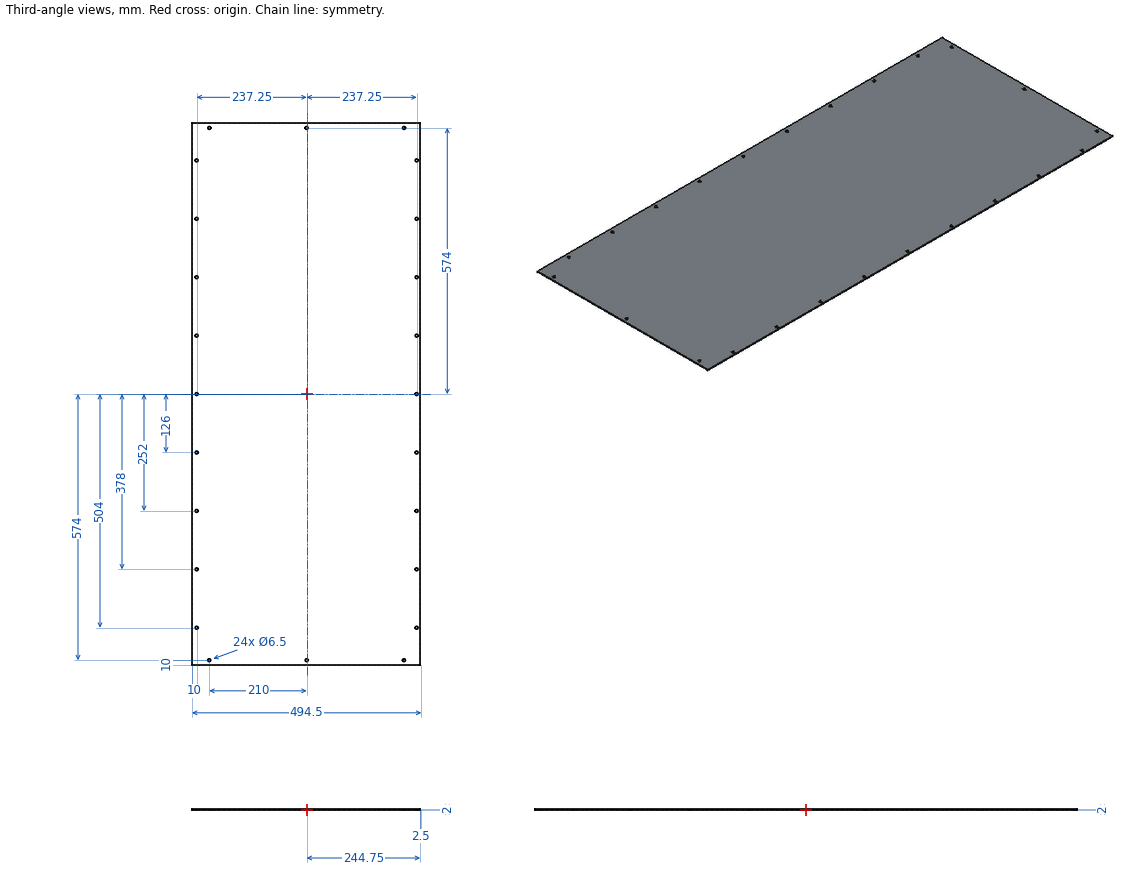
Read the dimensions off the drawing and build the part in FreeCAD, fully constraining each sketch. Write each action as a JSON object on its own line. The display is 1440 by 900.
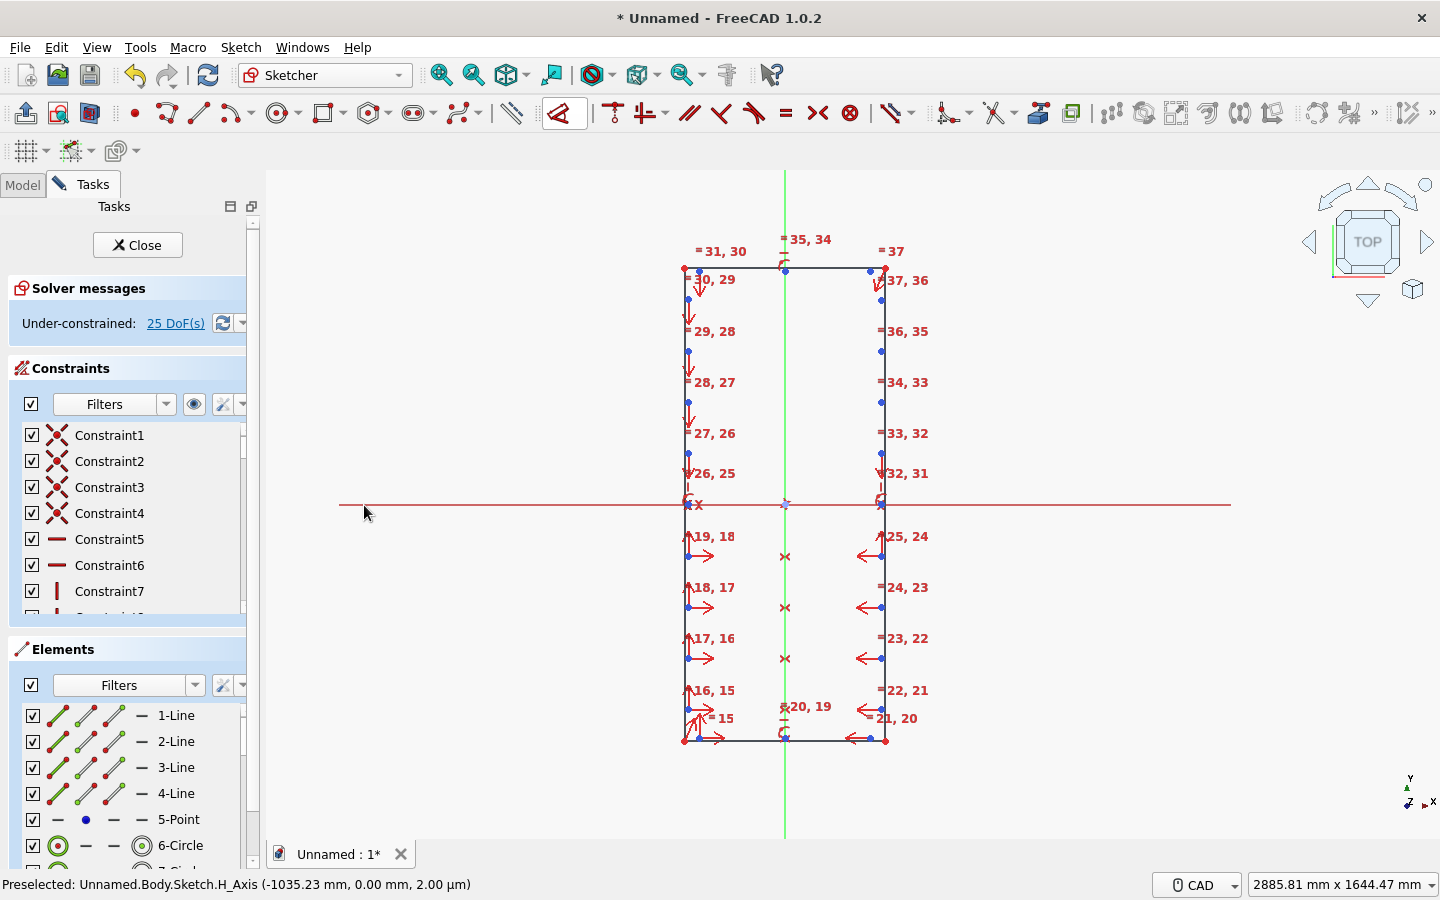
{"action": "left_click", "coordinate": [882, 608]}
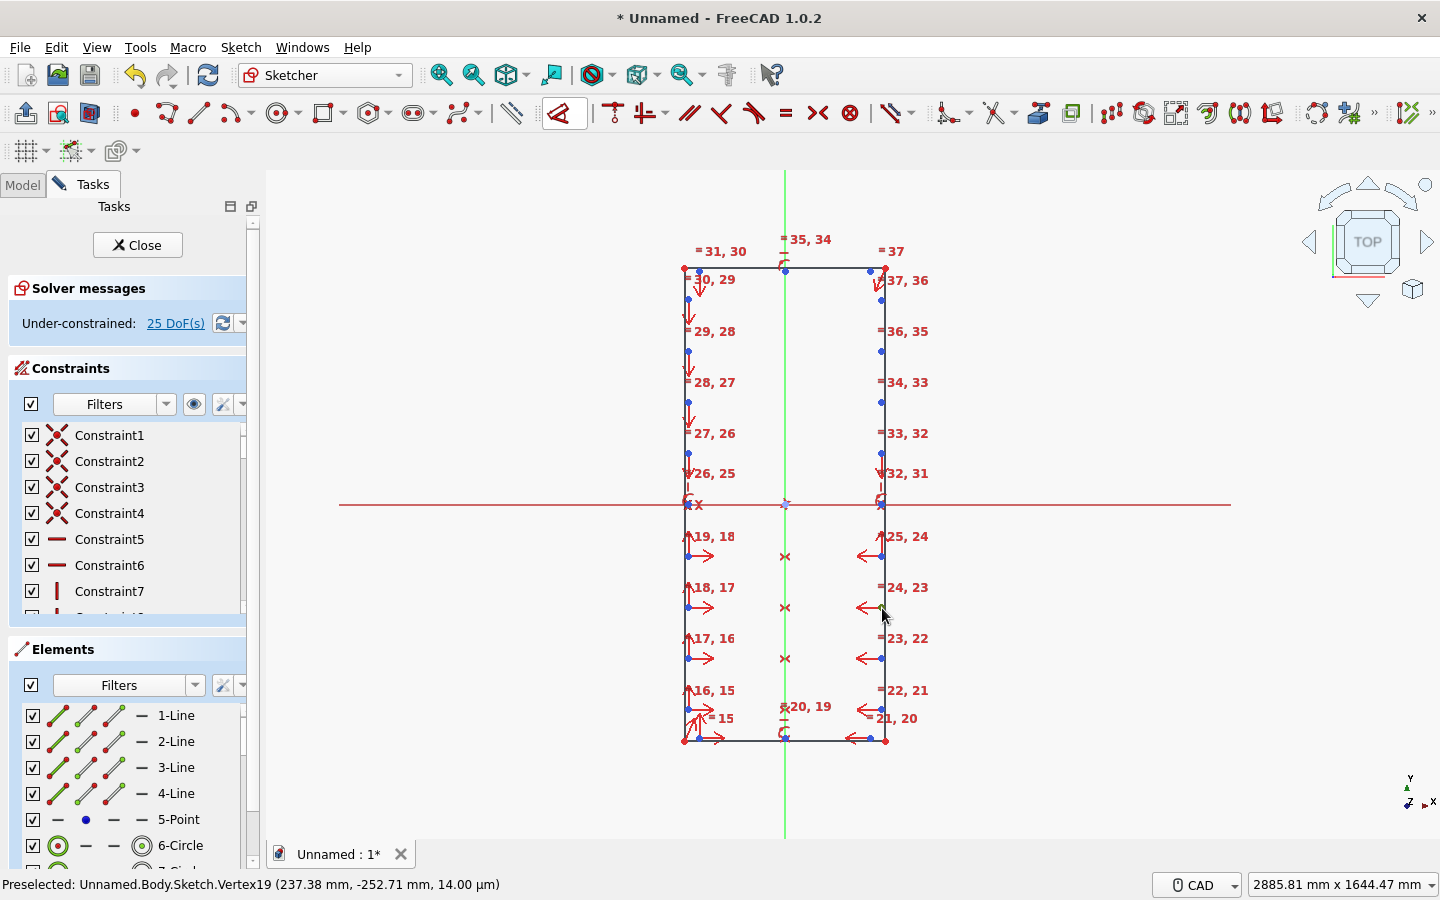
{"action": "left_click", "coordinate": [882, 403]}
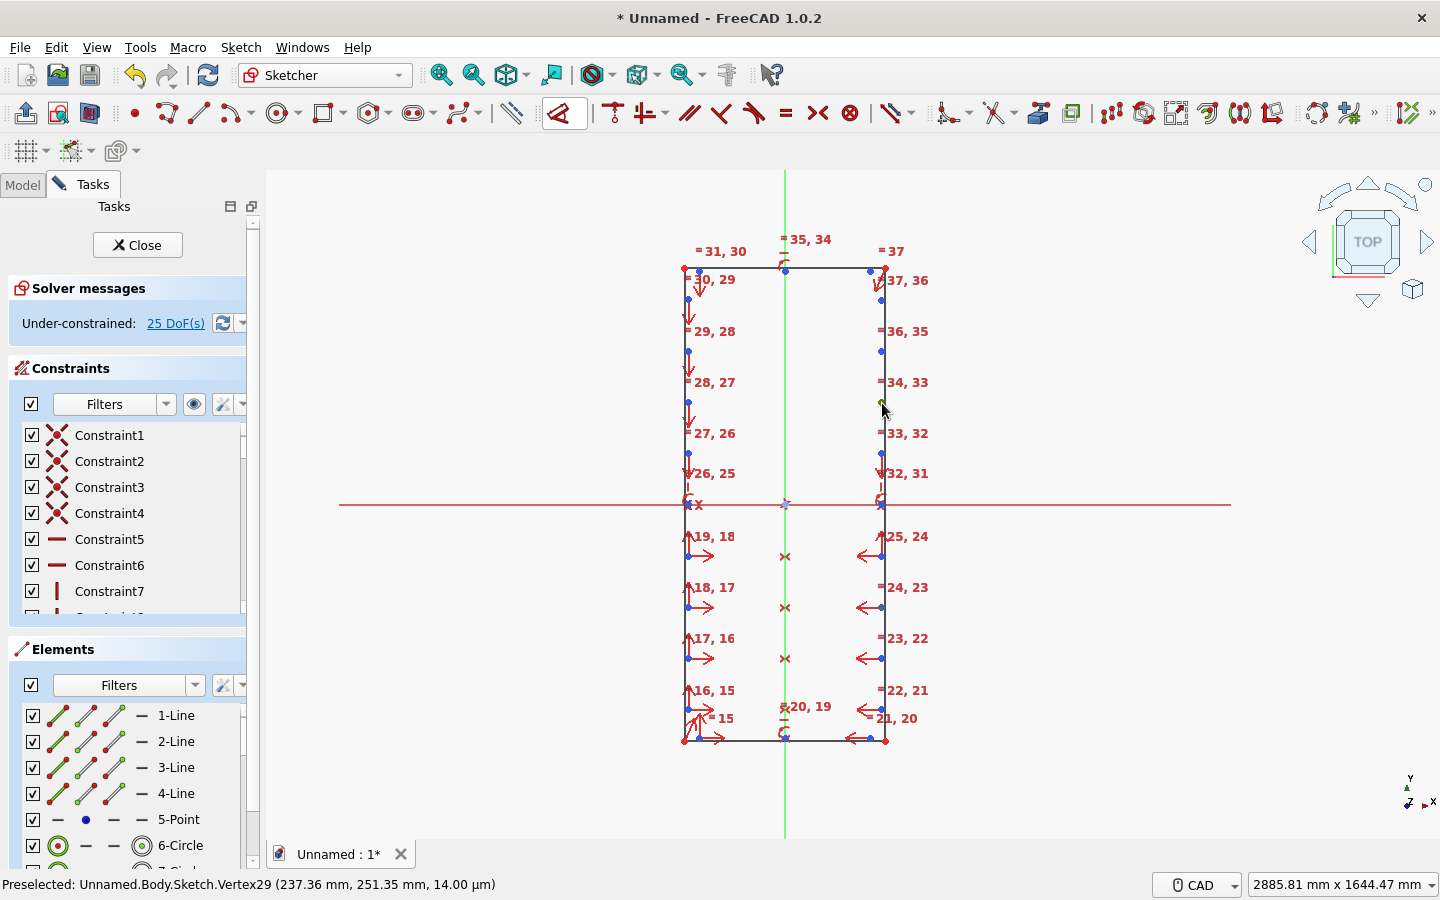
{"action": "left_click", "coordinate": [364, 505]}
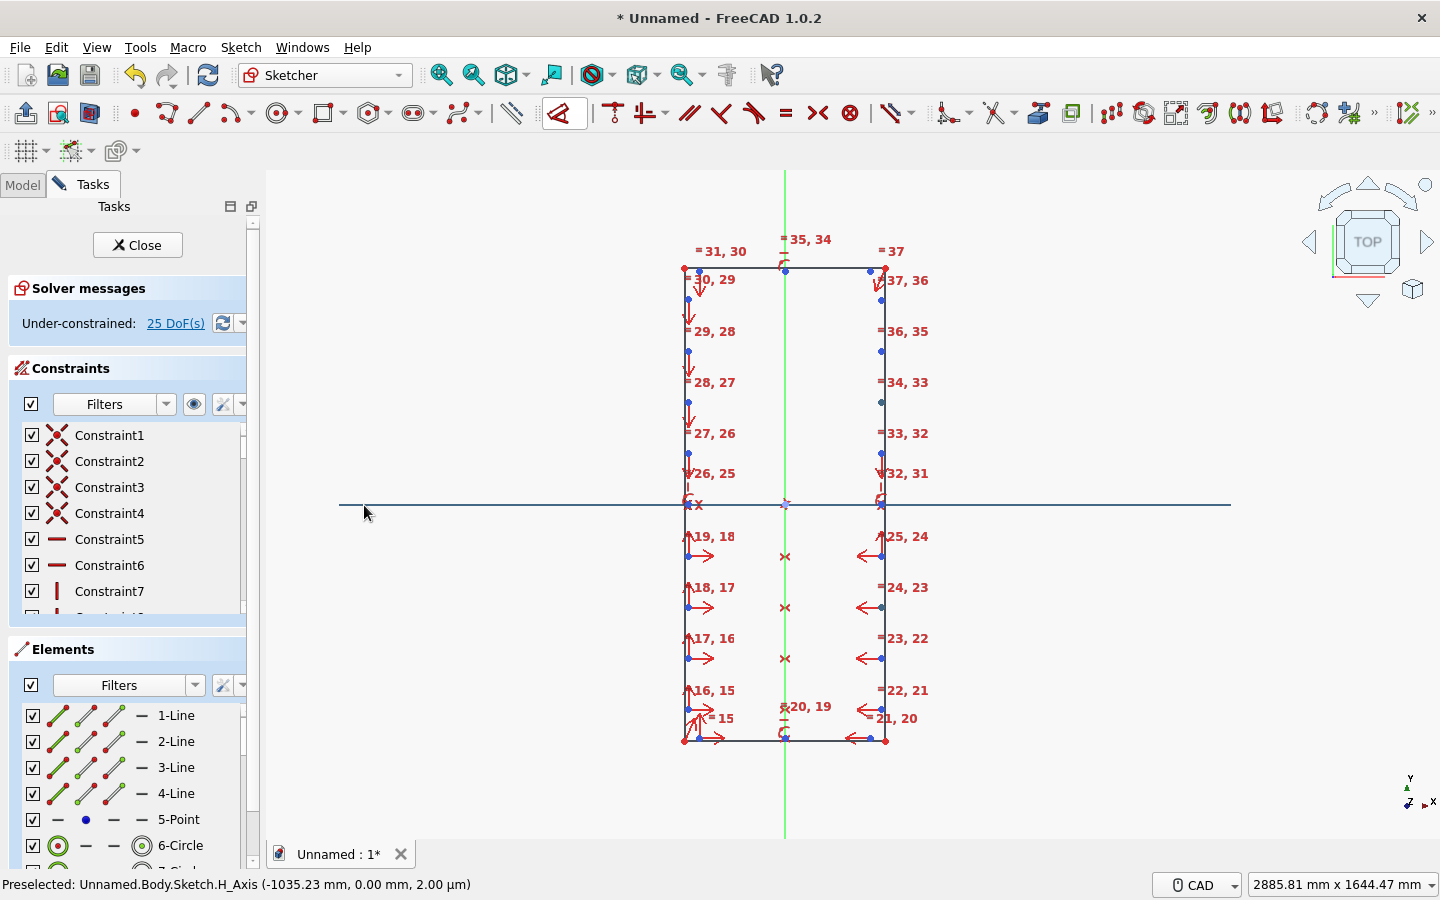
{"action": "key", "text": "s"}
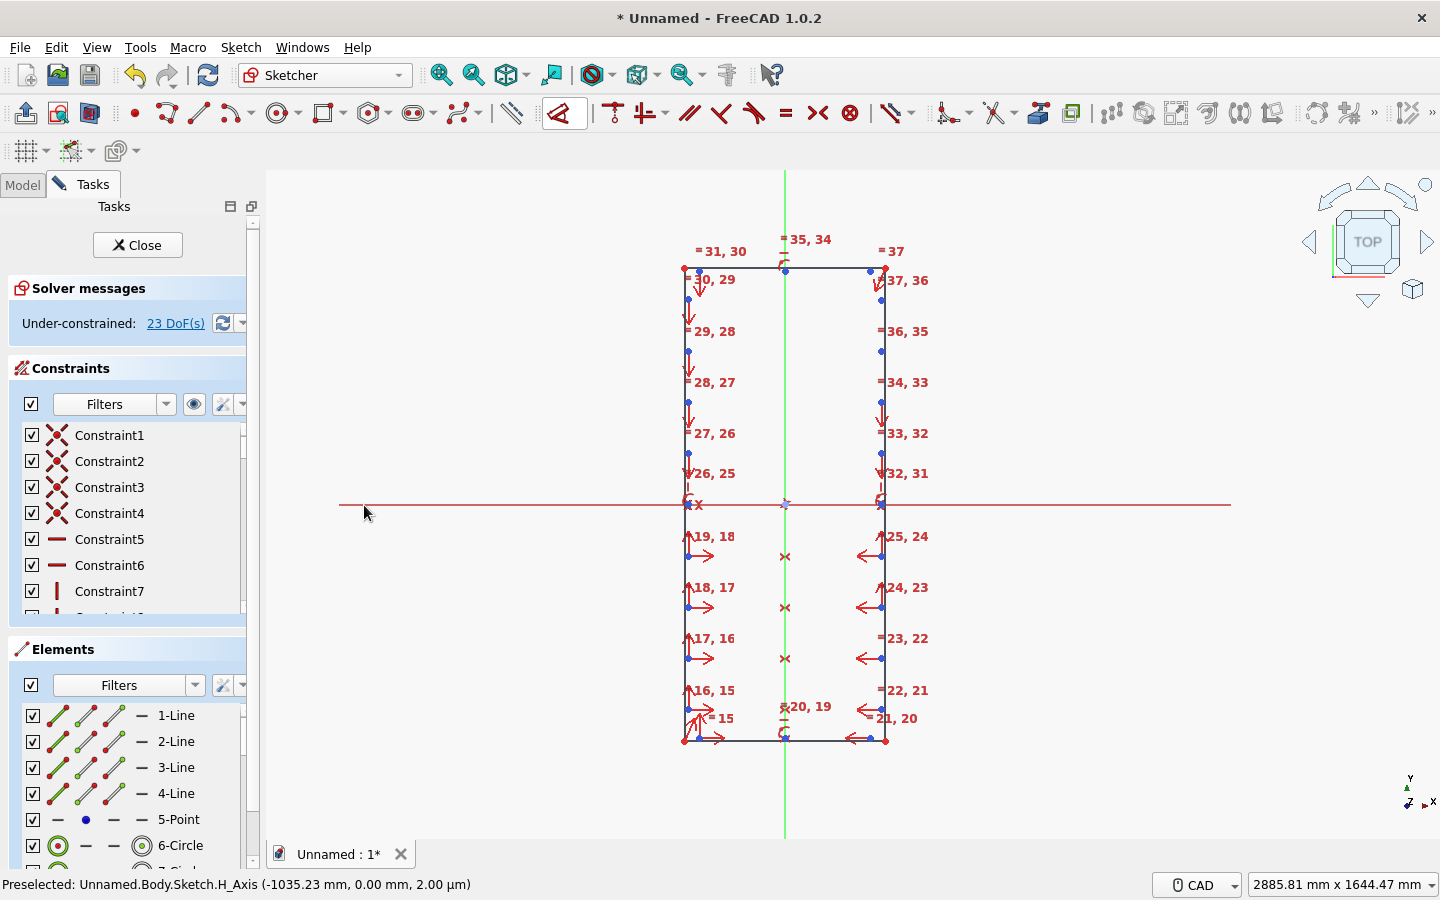
{"action": "left_click", "coordinate": [882, 659]}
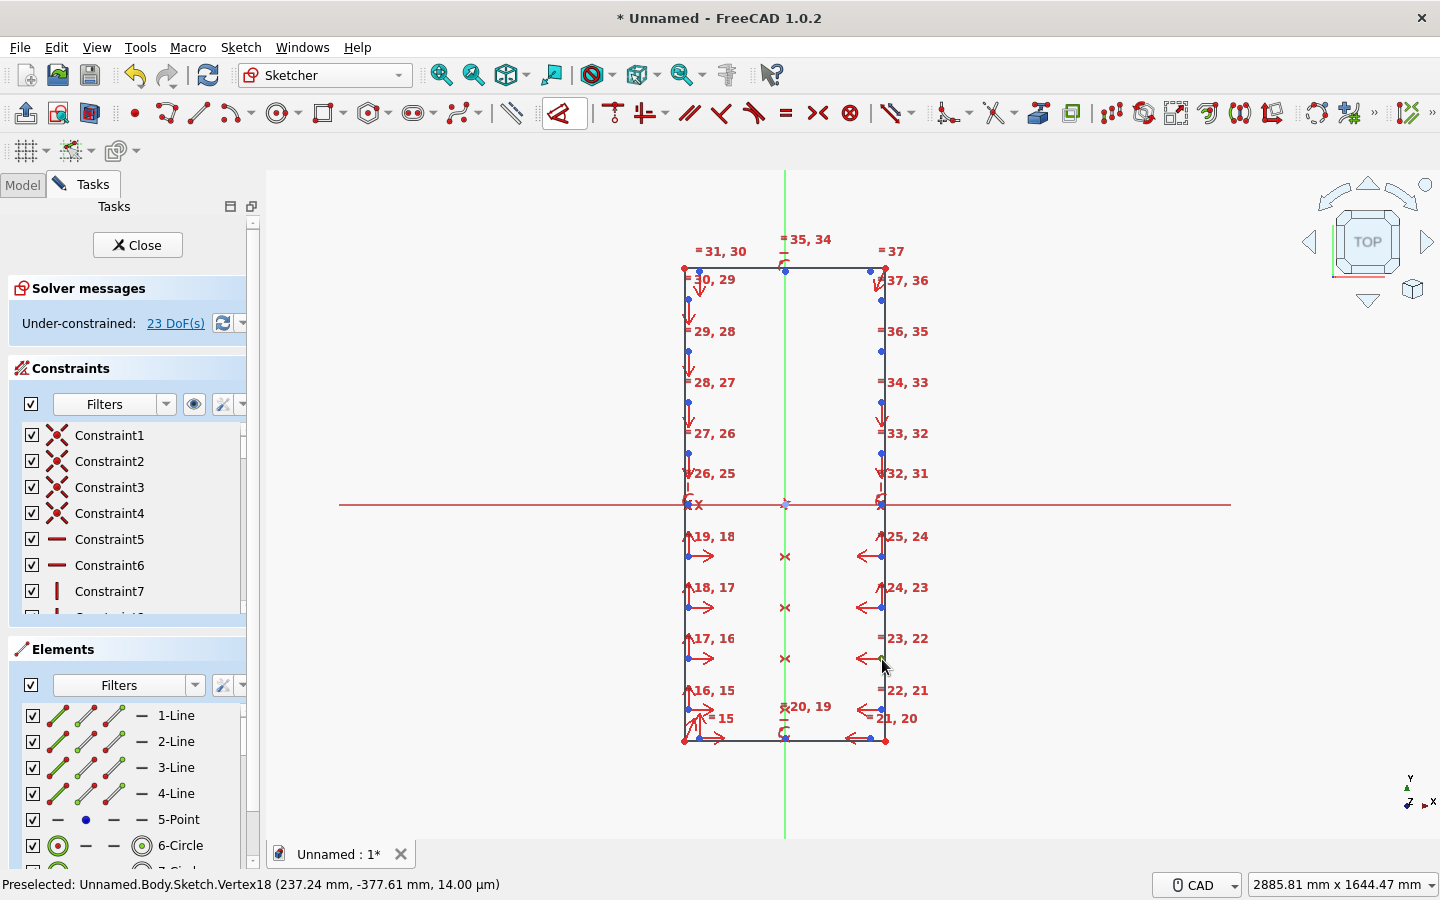
{"action": "left_click", "coordinate": [882, 351]}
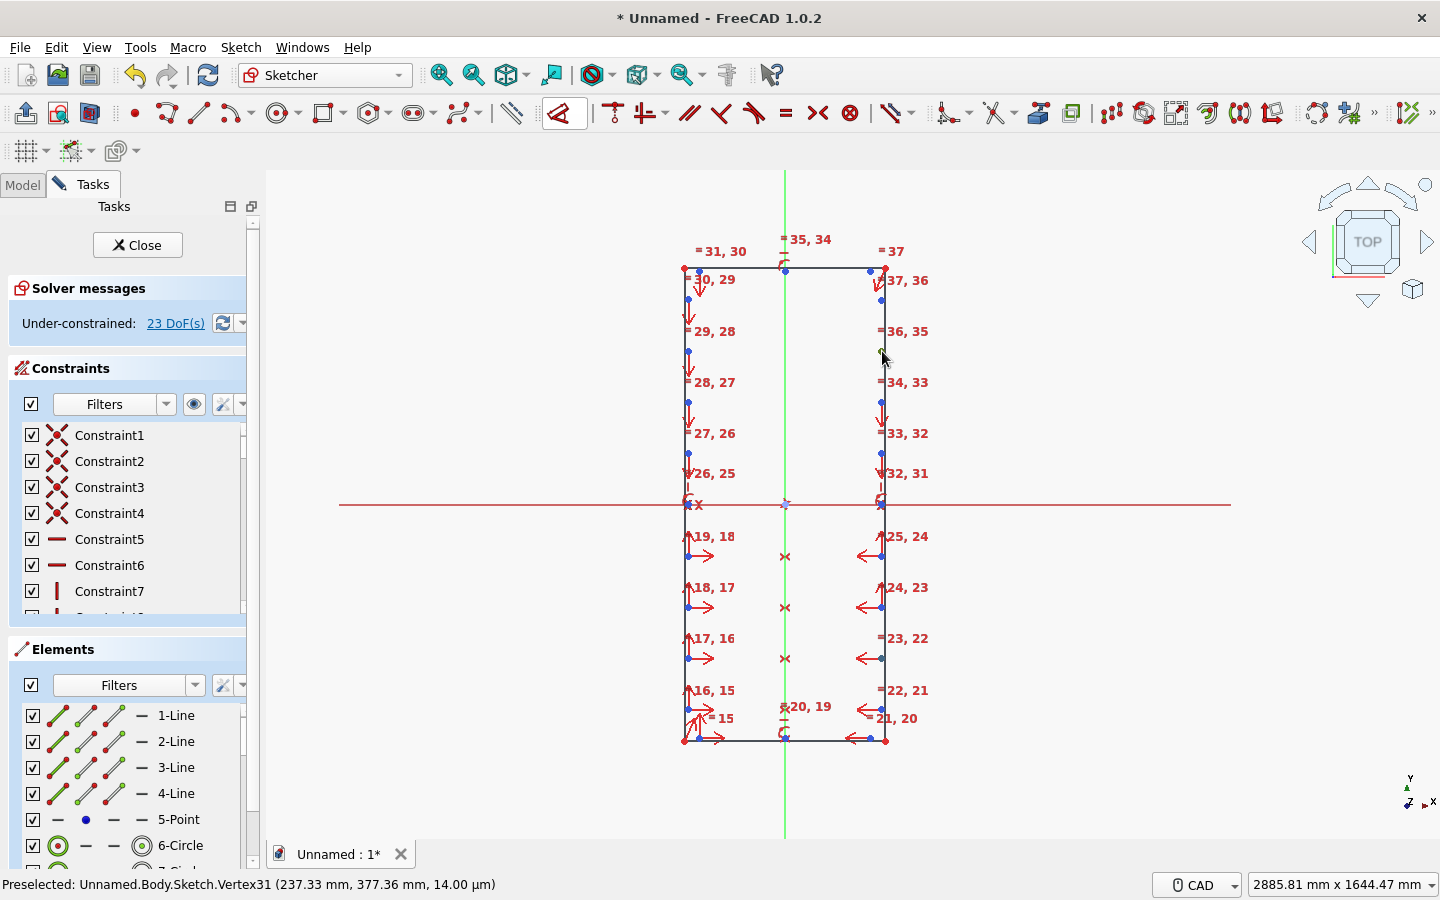
{"action": "left_click", "coordinate": [364, 505]}